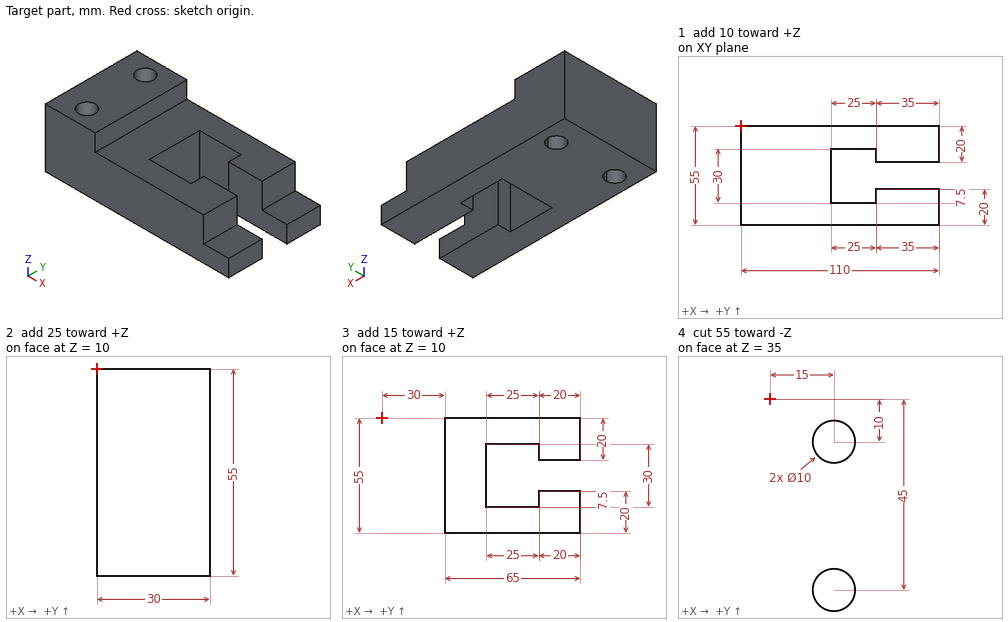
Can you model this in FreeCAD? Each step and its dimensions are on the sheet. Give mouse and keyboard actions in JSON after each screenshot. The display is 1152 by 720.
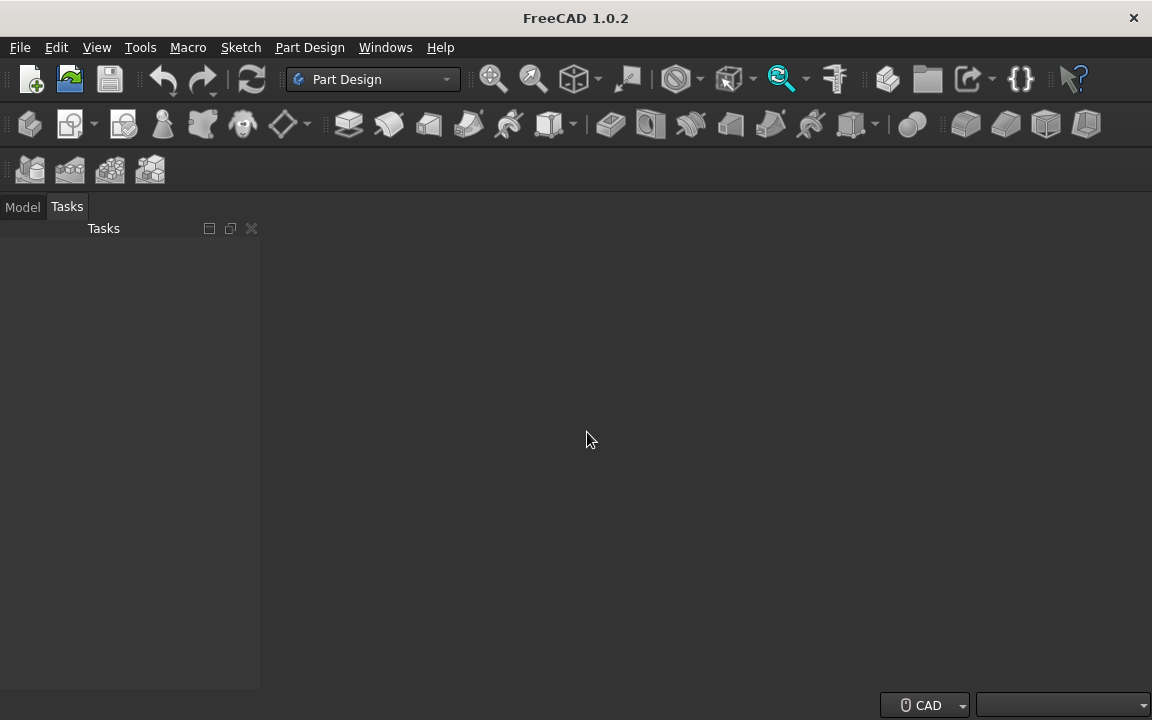
{"action": "left_click", "coordinate": [30, 80]}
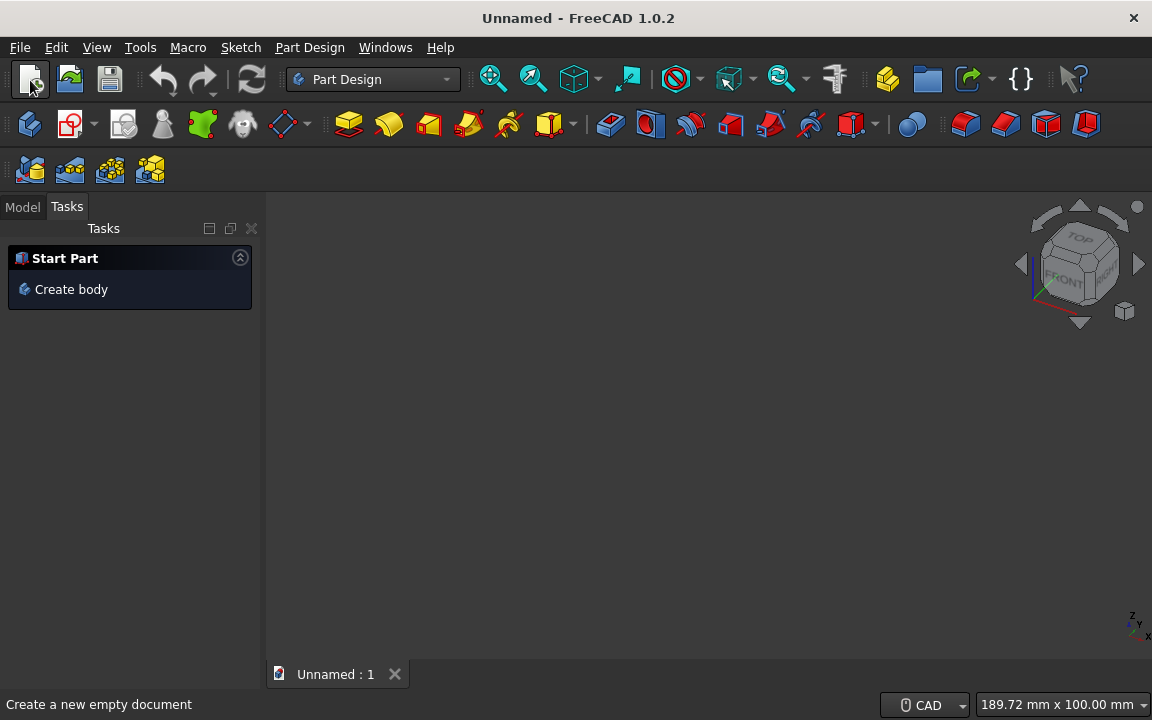
{"action": "left_click", "coordinate": [70, 124]}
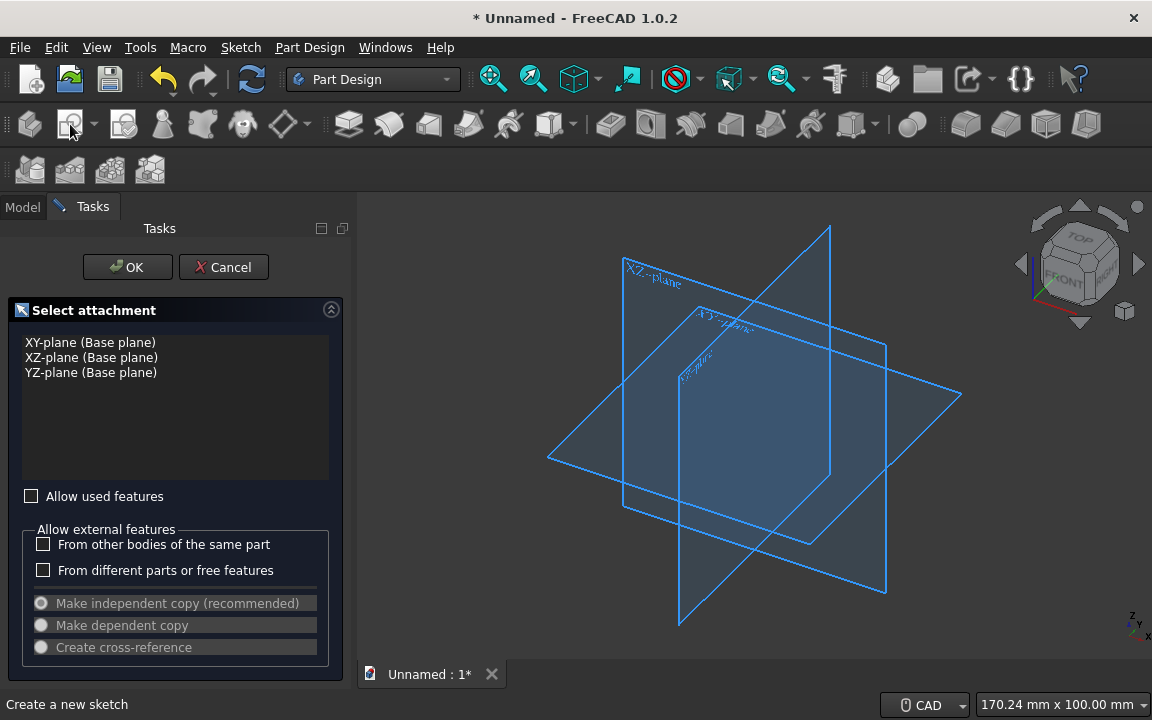
{"action": "left_click", "coordinate": [82, 342]}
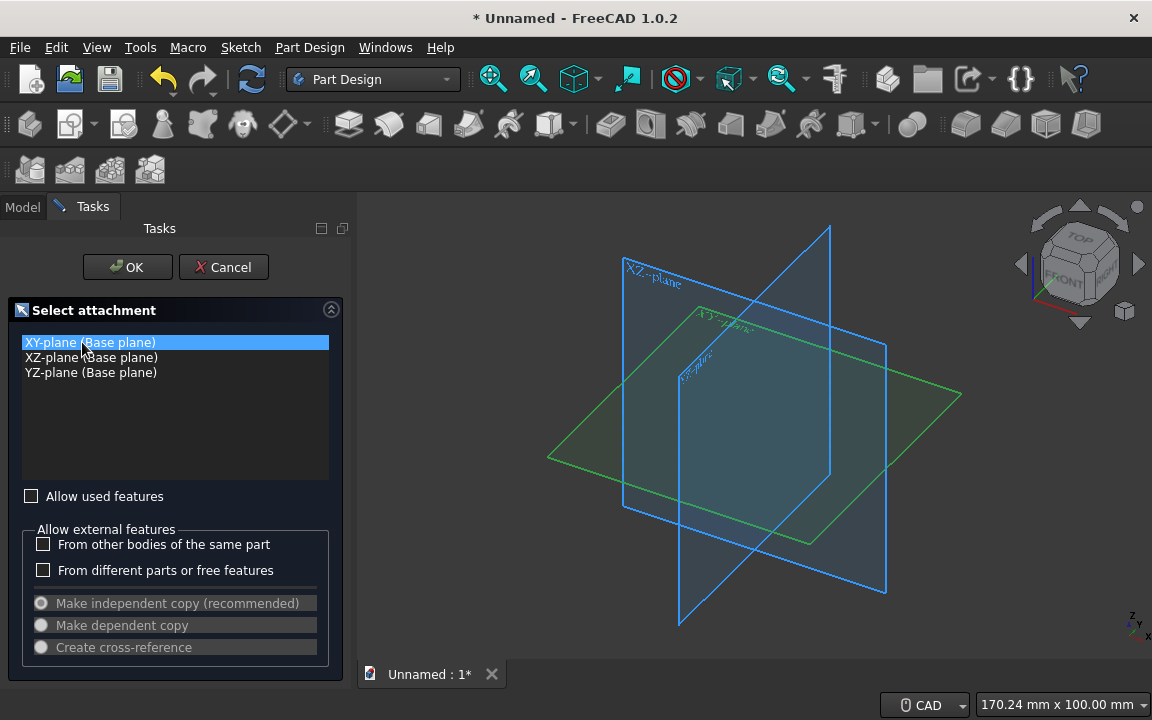
{"action": "left_click", "coordinate": [128, 267]}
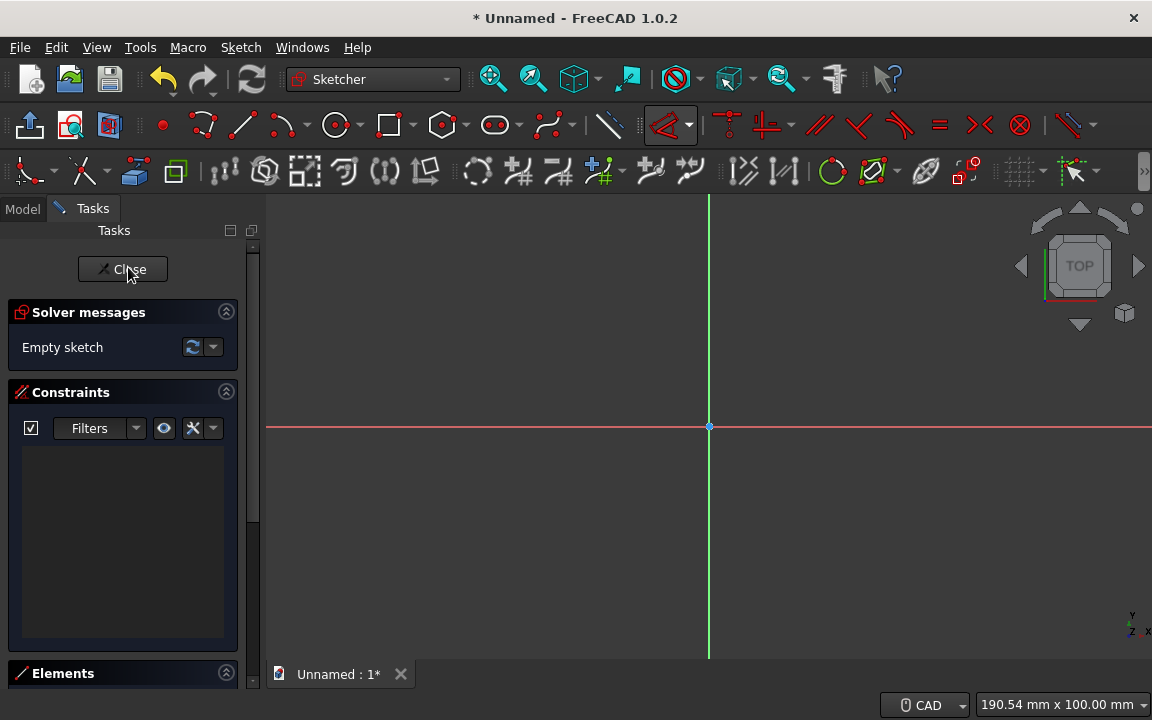
{"action": "scroll", "coordinate": [294, 222], "scroll_direction": "down", "scroll_amount": 2}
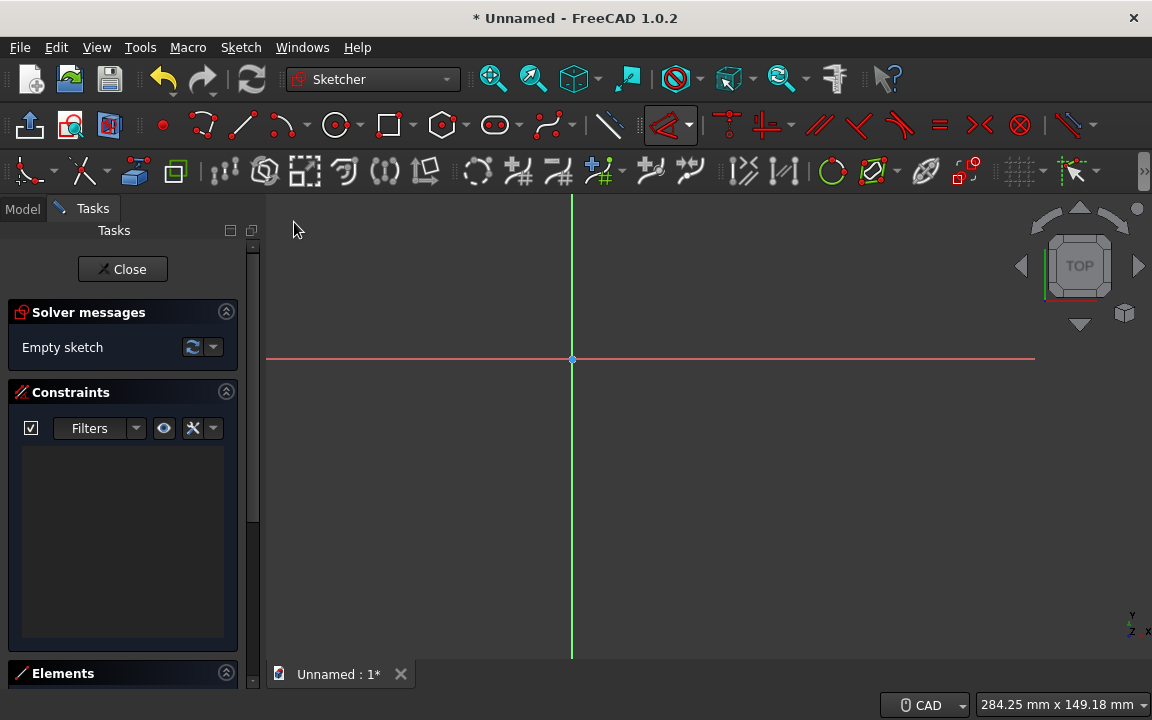
{"action": "scroll", "coordinate": [953, 482], "scroll_direction": "up", "scroll_amount": 2}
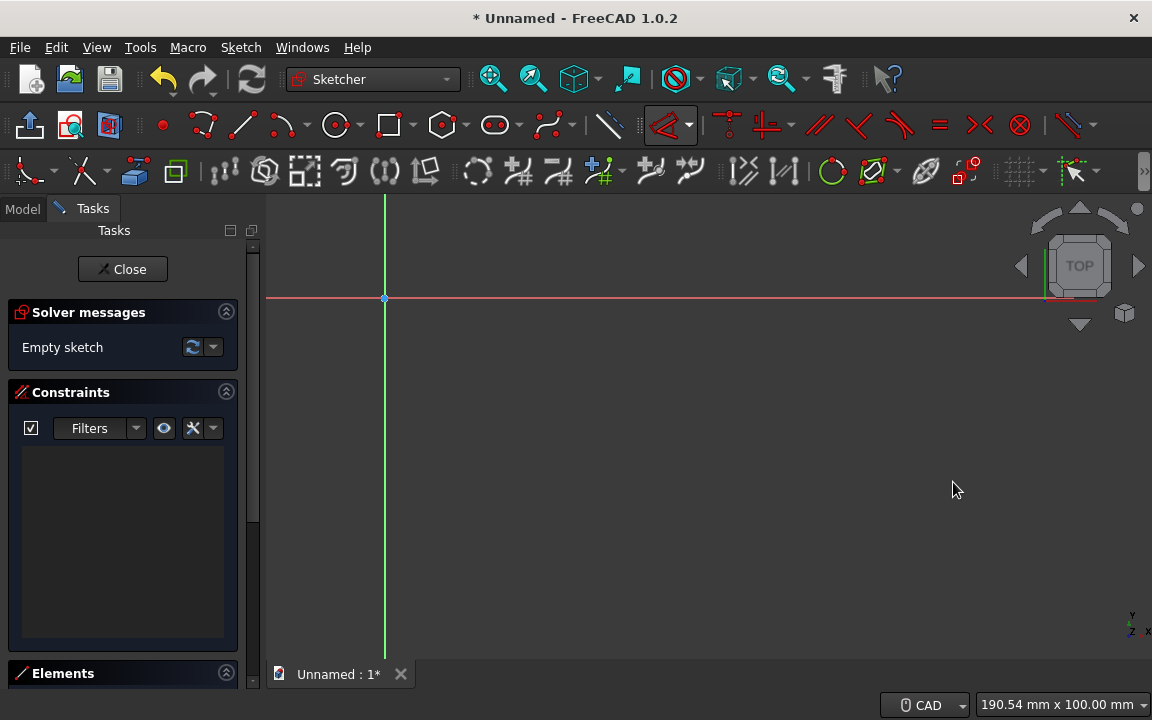
{"action": "left_click", "coordinate": [204, 126]}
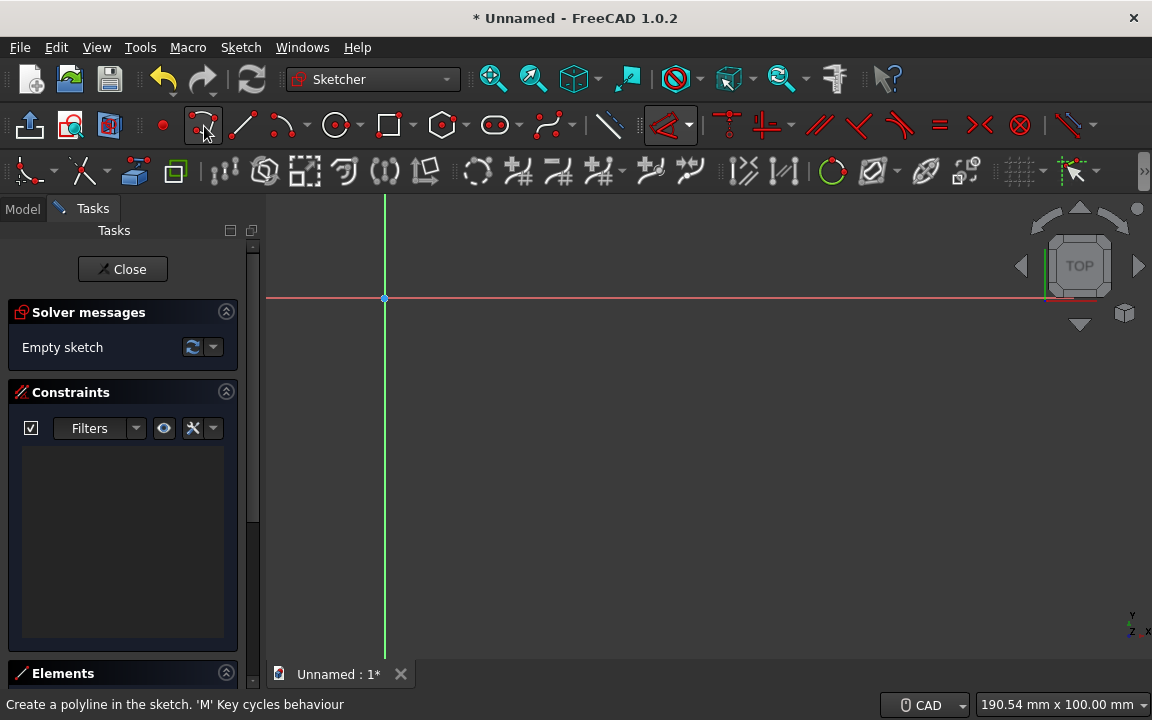
{"action": "left_click", "coordinate": [385, 298]}
{"action": "left_click", "coordinate": [394, 554]}
{"action": "left_click", "coordinate": [896, 554]}
{"action": "left_click", "coordinate": [896, 461]}
{"action": "left_click", "coordinate": [733, 461]}
{"action": "left_click", "coordinate": [733, 496]}
{"action": "left_click", "coordinate": [617, 496]}
{"action": "left_click", "coordinate": [617, 356]}
{"action": "left_click", "coordinate": [733, 356]}
{"action": "left_click", "coordinate": [733, 391]}
{"action": "left_click", "coordinate": [896, 391]}
{"action": "left_click", "coordinate": [896, 307]}
{"action": "left_click", "coordinate": [385, 298]}
{"action": "key", "text": "Escape"}
{"action": "key", "text": "Escape"}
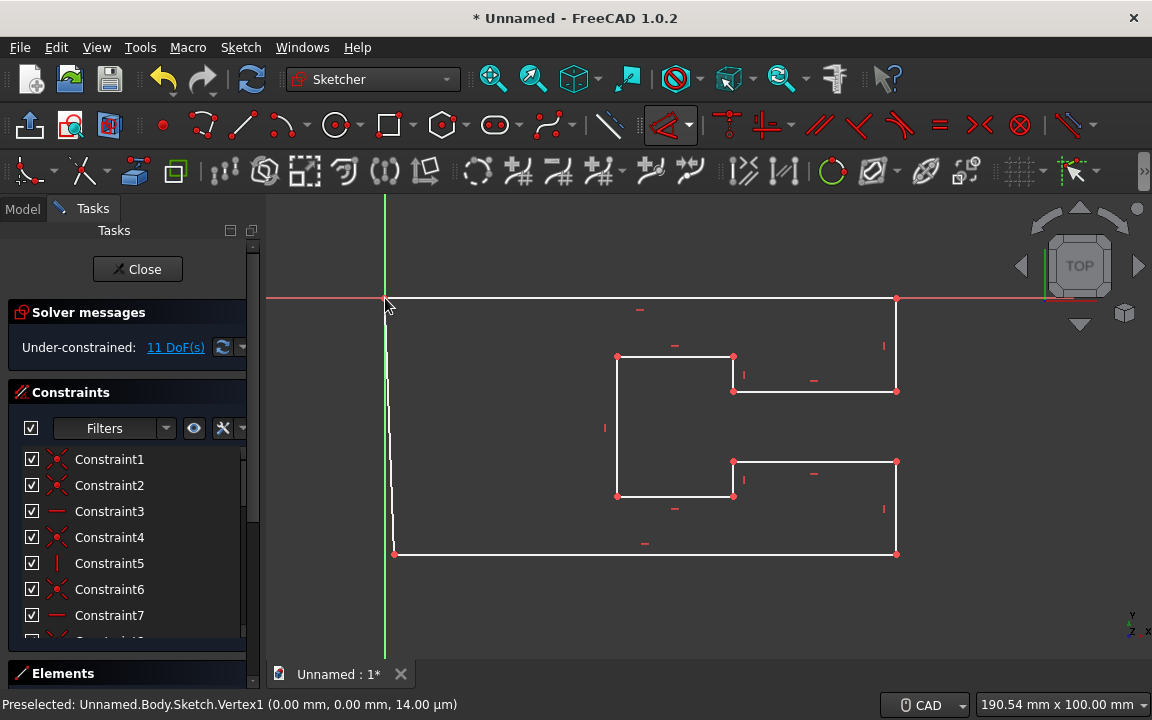
{"action": "left_click", "coordinate": [387, 375]}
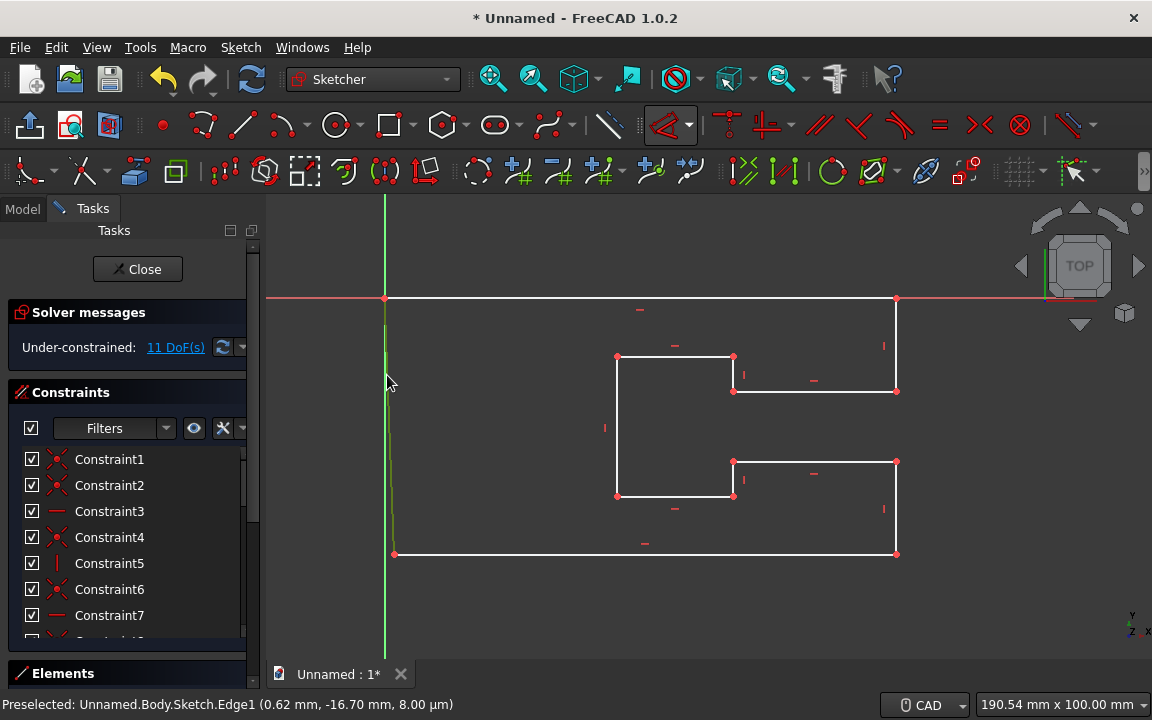
{"action": "left_click", "coordinate": [794, 126]}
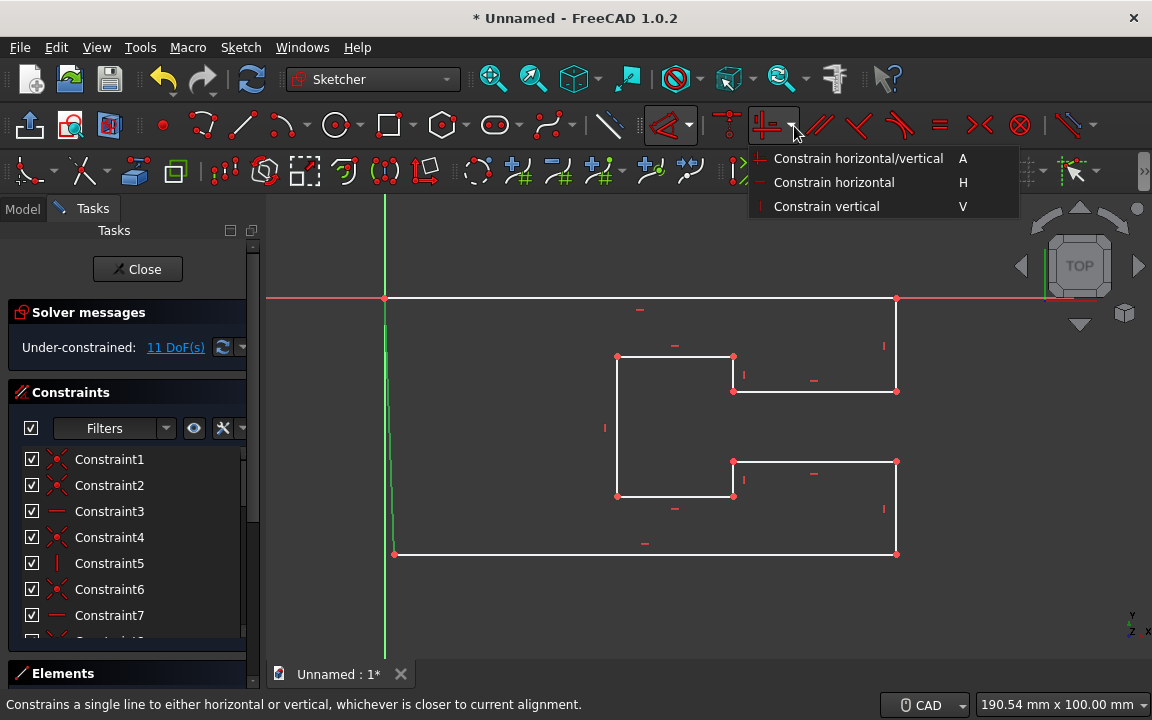
{"action": "left_click", "coordinate": [884, 206]}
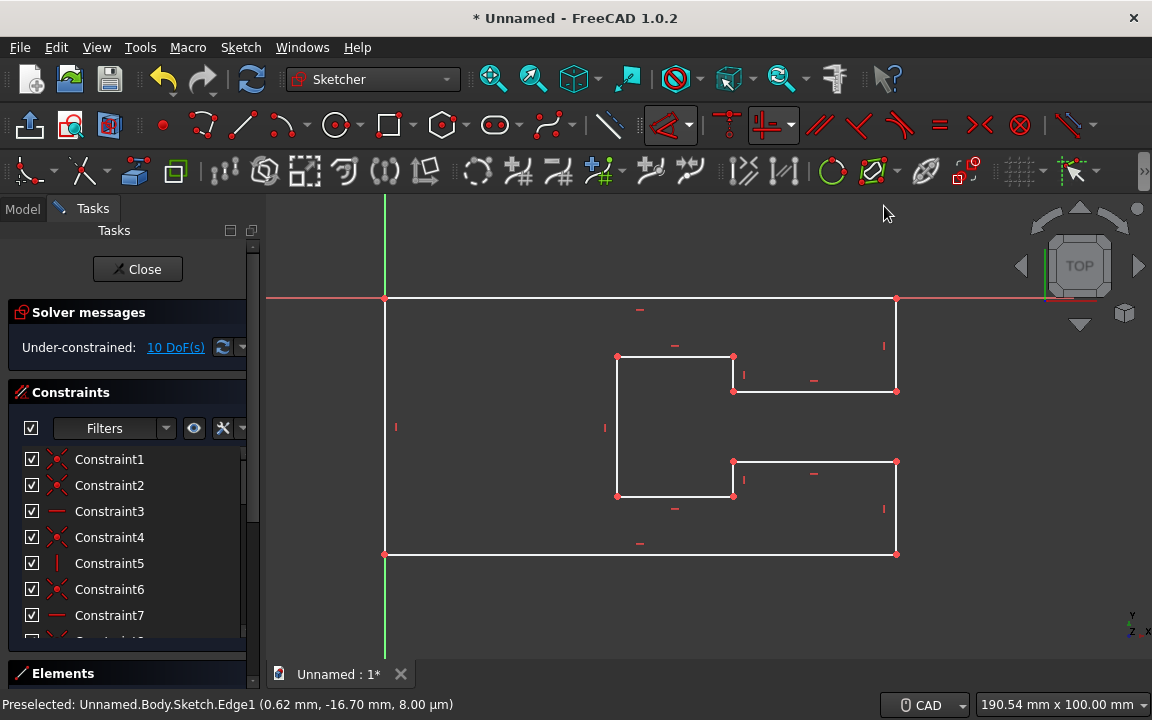
{"action": "left_click", "coordinate": [664, 126]}